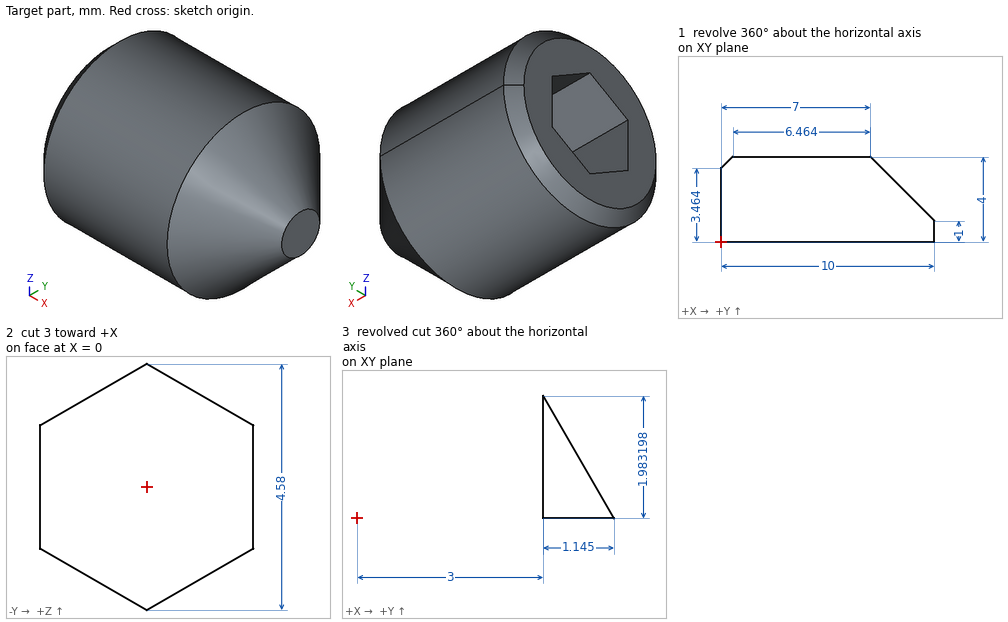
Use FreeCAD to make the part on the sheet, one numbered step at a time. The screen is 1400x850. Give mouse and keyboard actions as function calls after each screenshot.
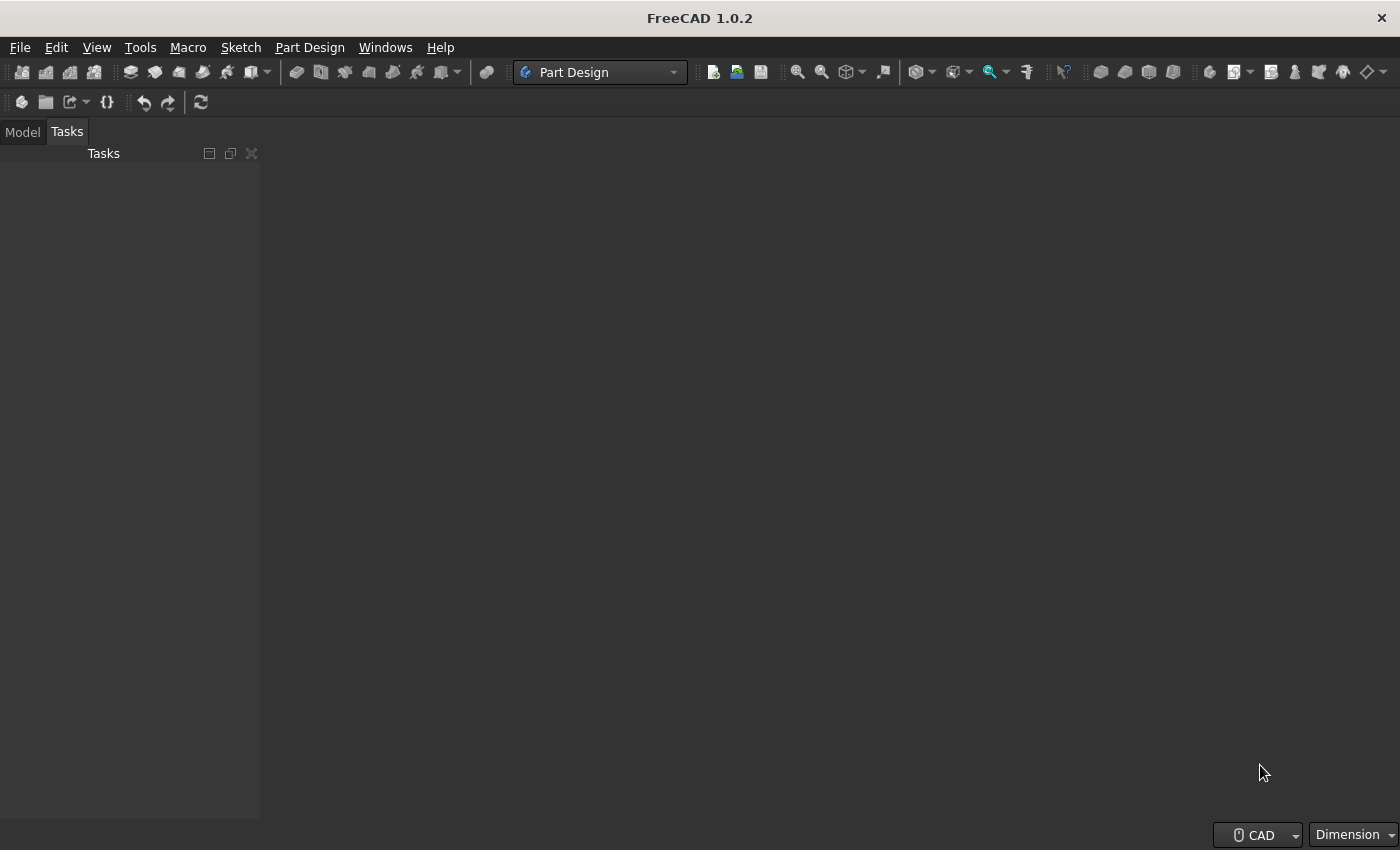
click(714, 72)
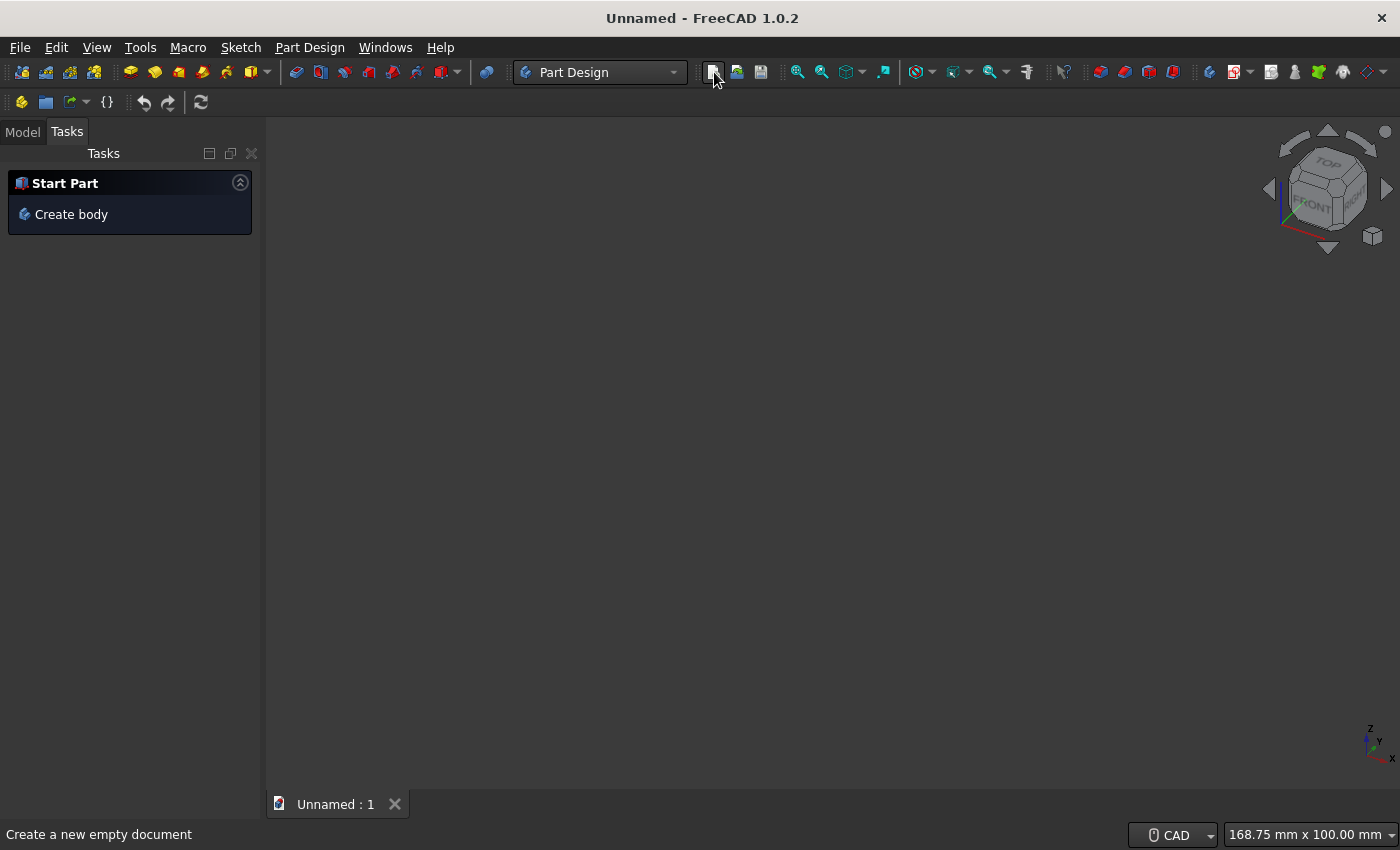
click(1234, 72)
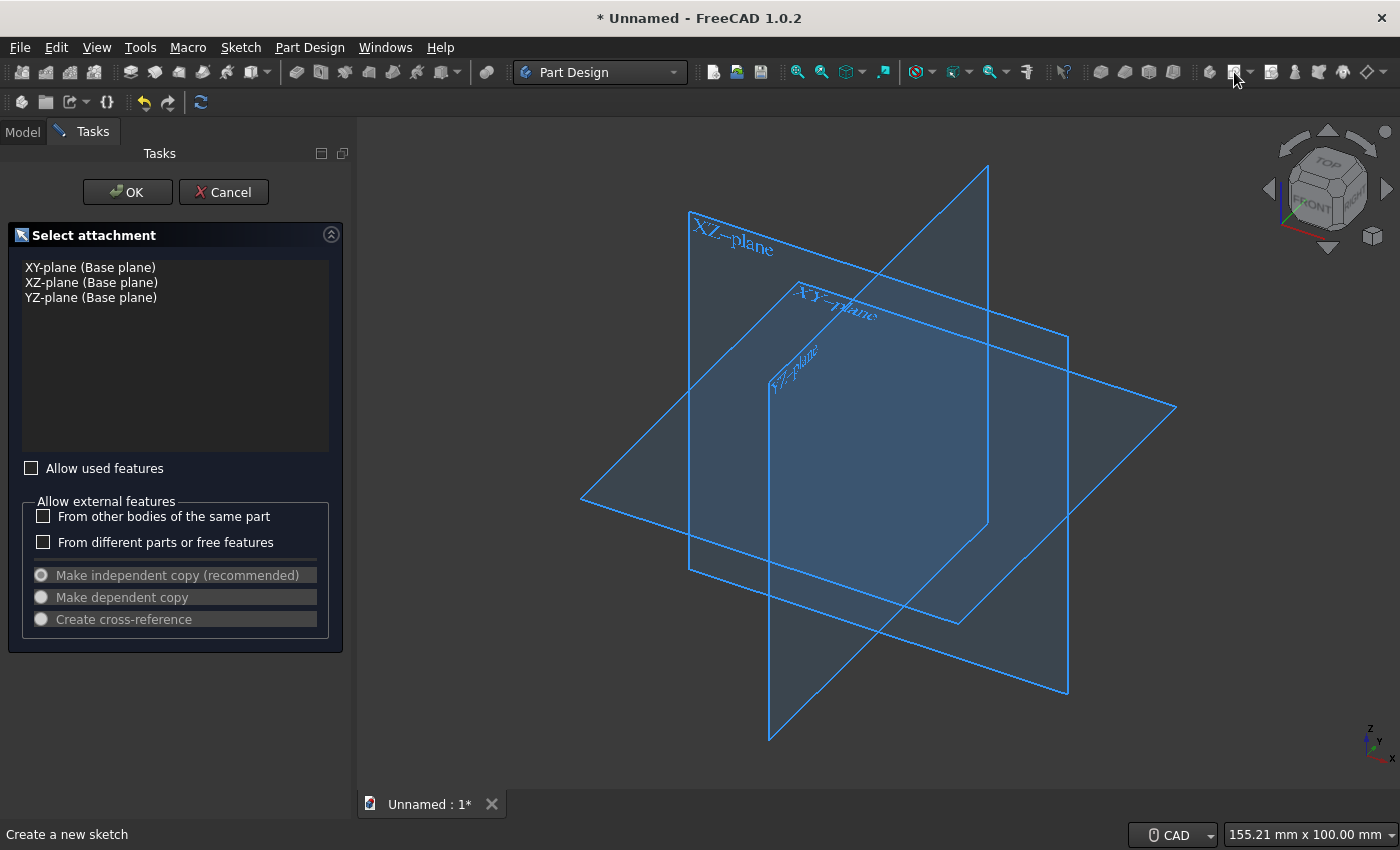
click(82, 268)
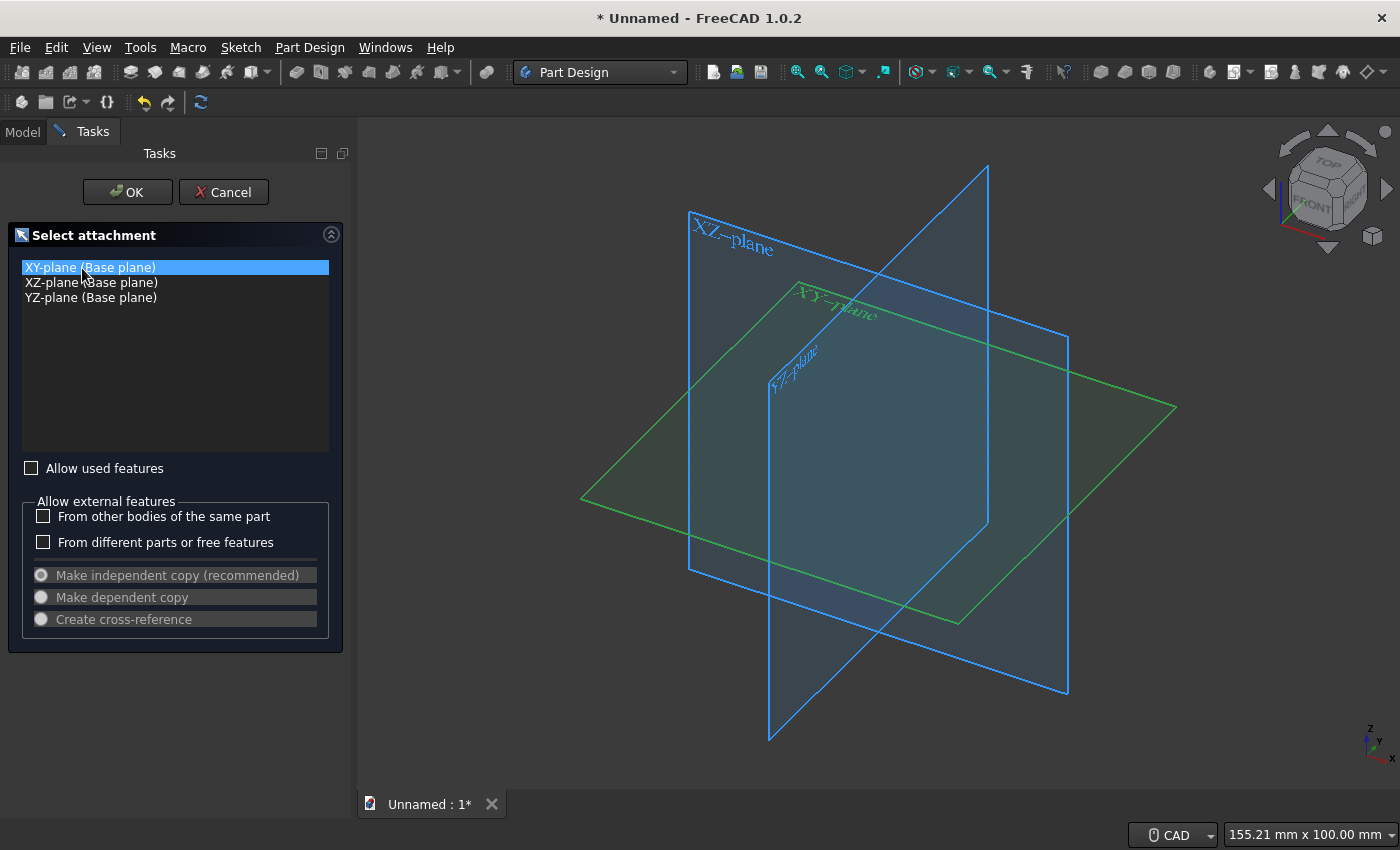
click(128, 192)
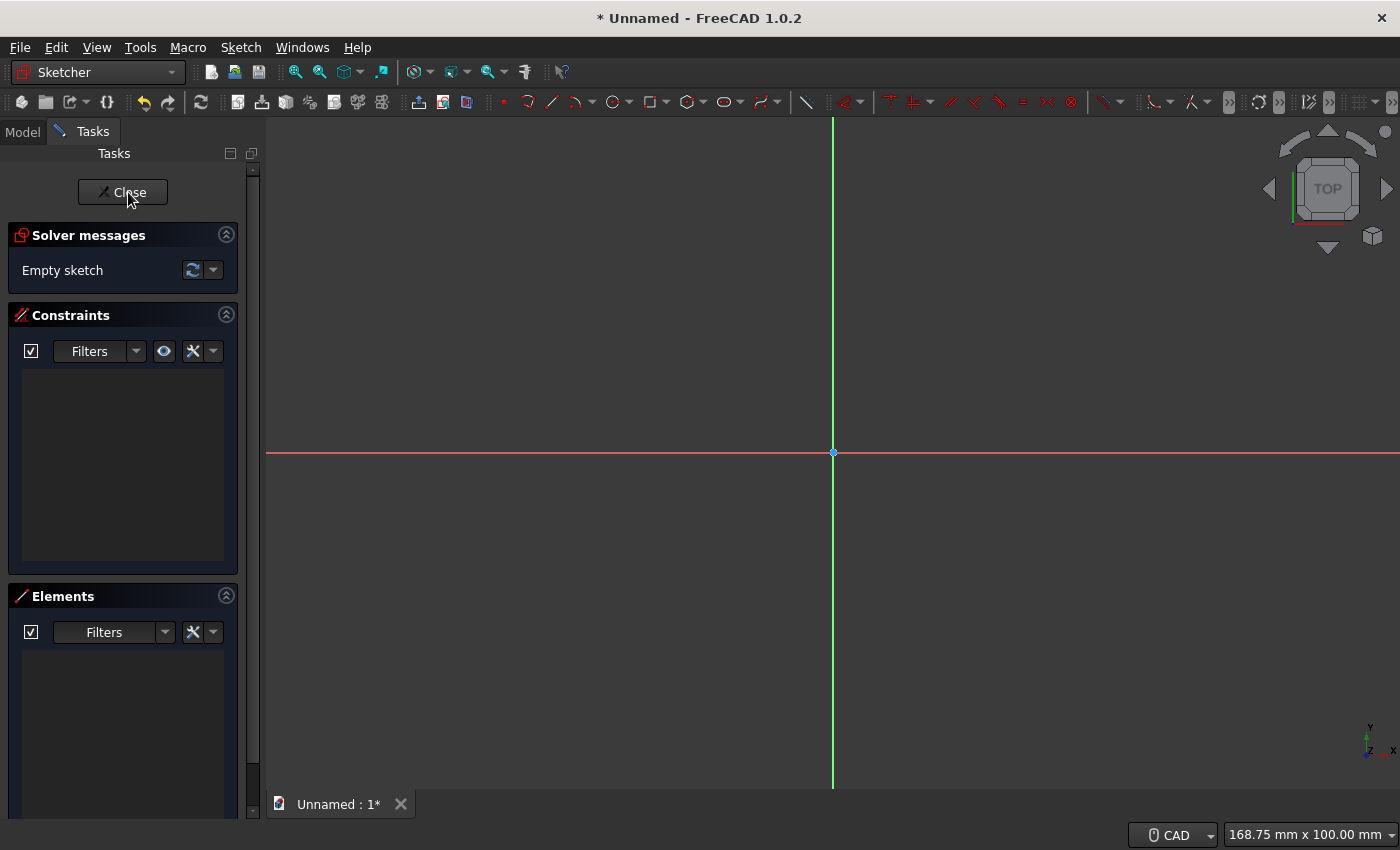
scroll(879, 438, up, 11)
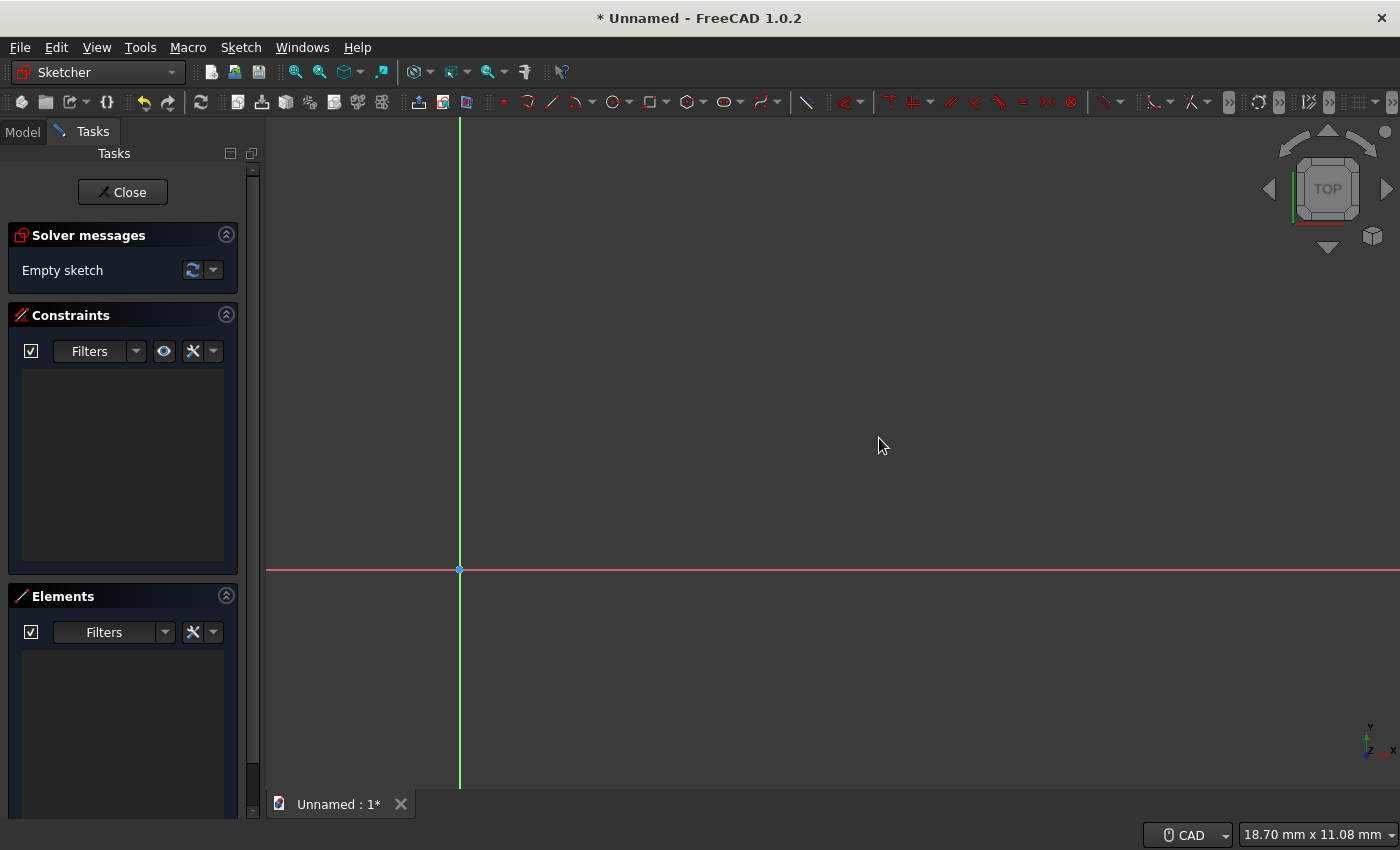
click(528, 102)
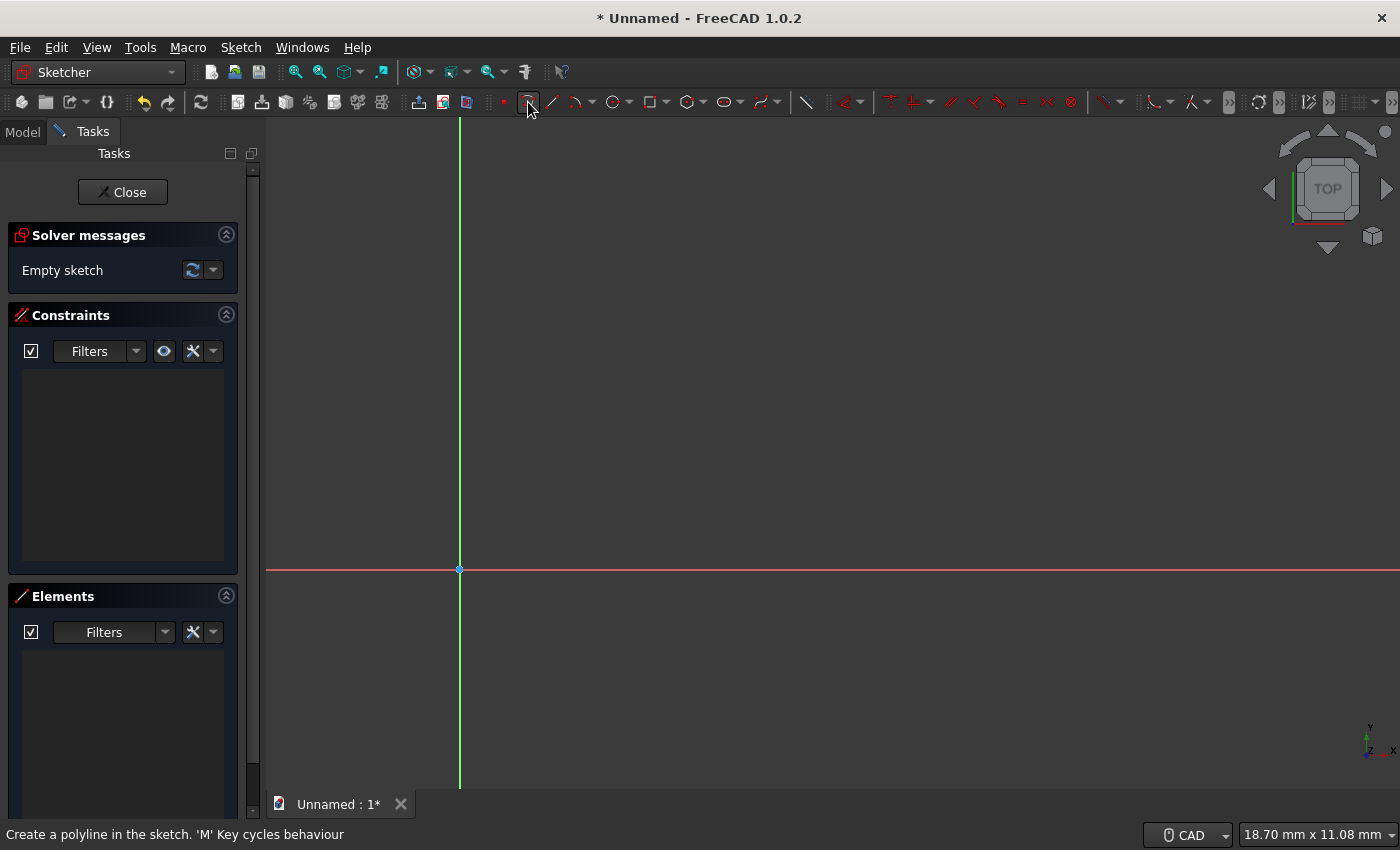
click(460, 570)
click(1066, 561)
click(1066, 509)
click(884, 327)
click(492, 327)
click(469, 359)
click(460, 570)
key(Escape)
key(Escape)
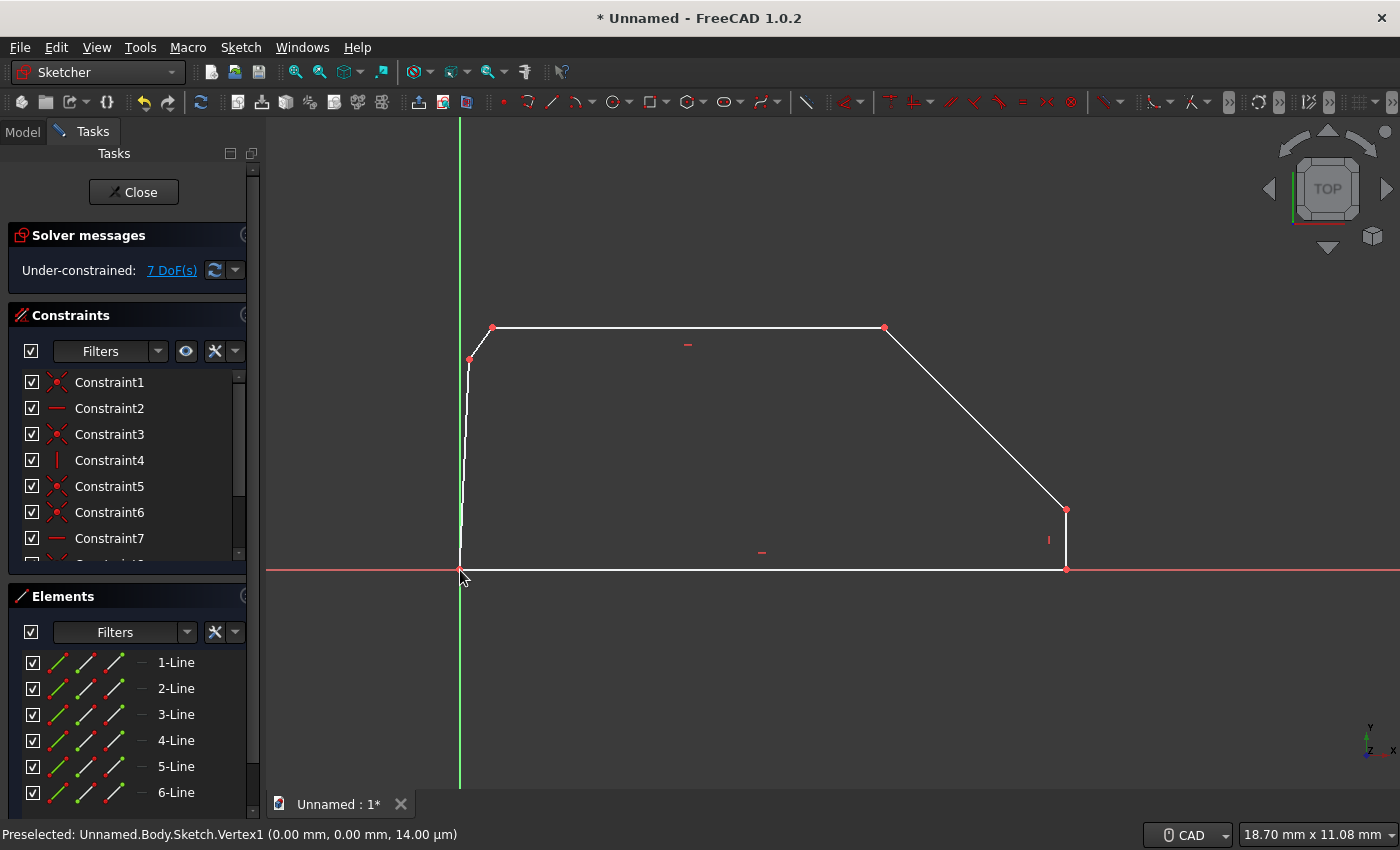
click(462, 507)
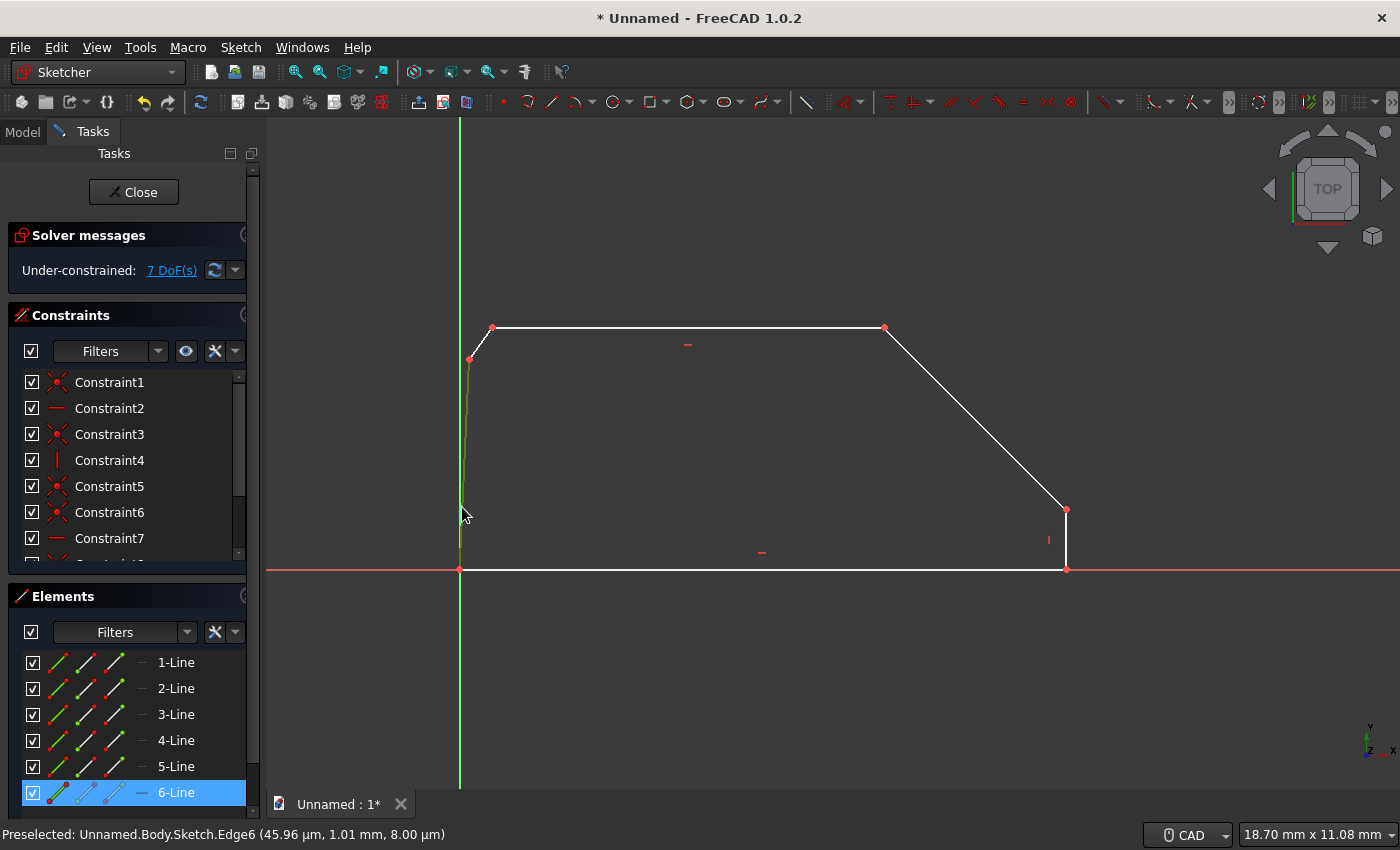
key(v)